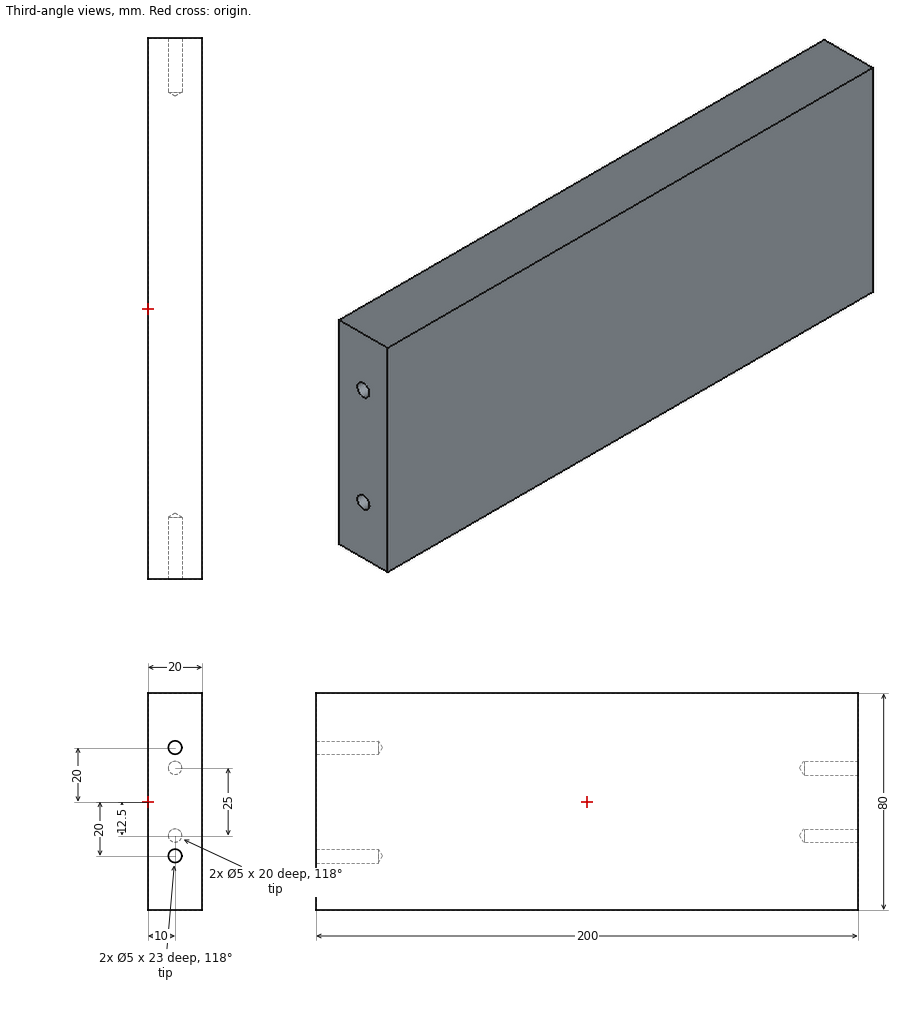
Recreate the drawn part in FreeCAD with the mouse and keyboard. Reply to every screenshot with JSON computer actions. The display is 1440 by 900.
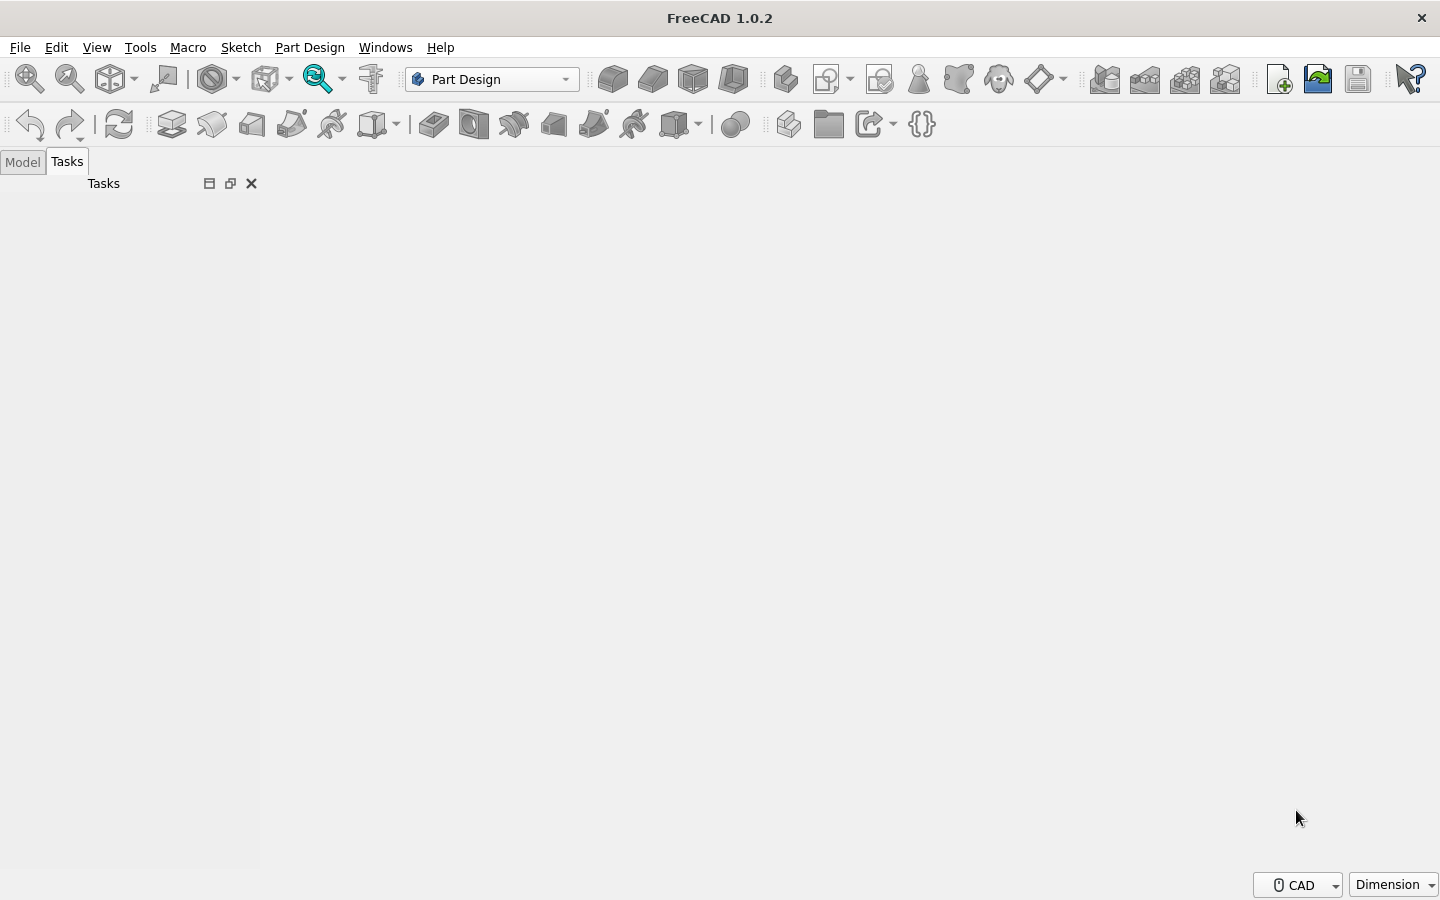
{"action": "left_click", "coordinate": [1278, 80]}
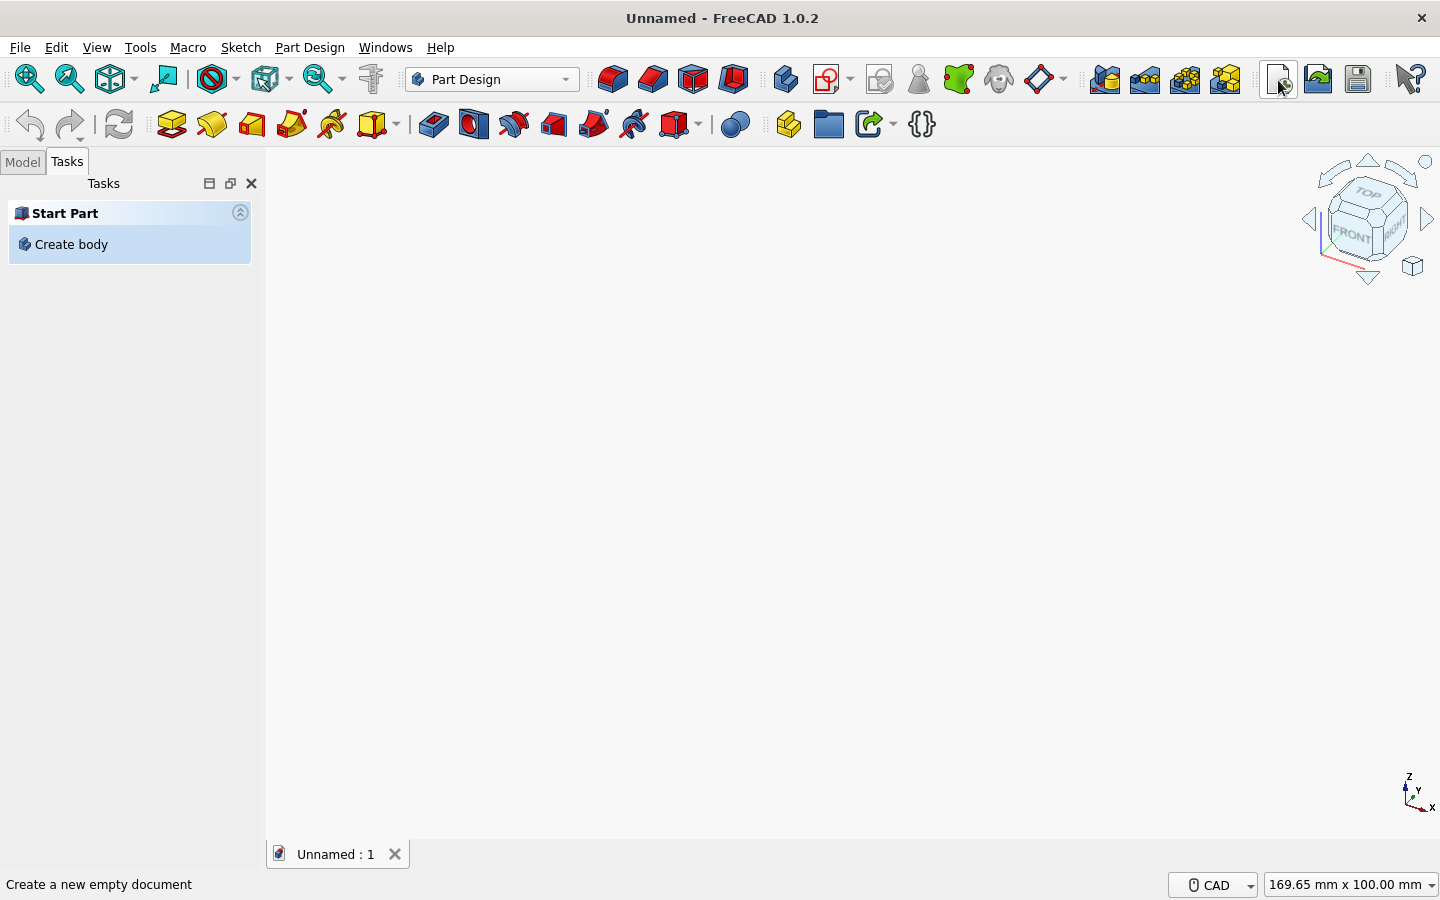
{"action": "left_click", "coordinate": [826, 80]}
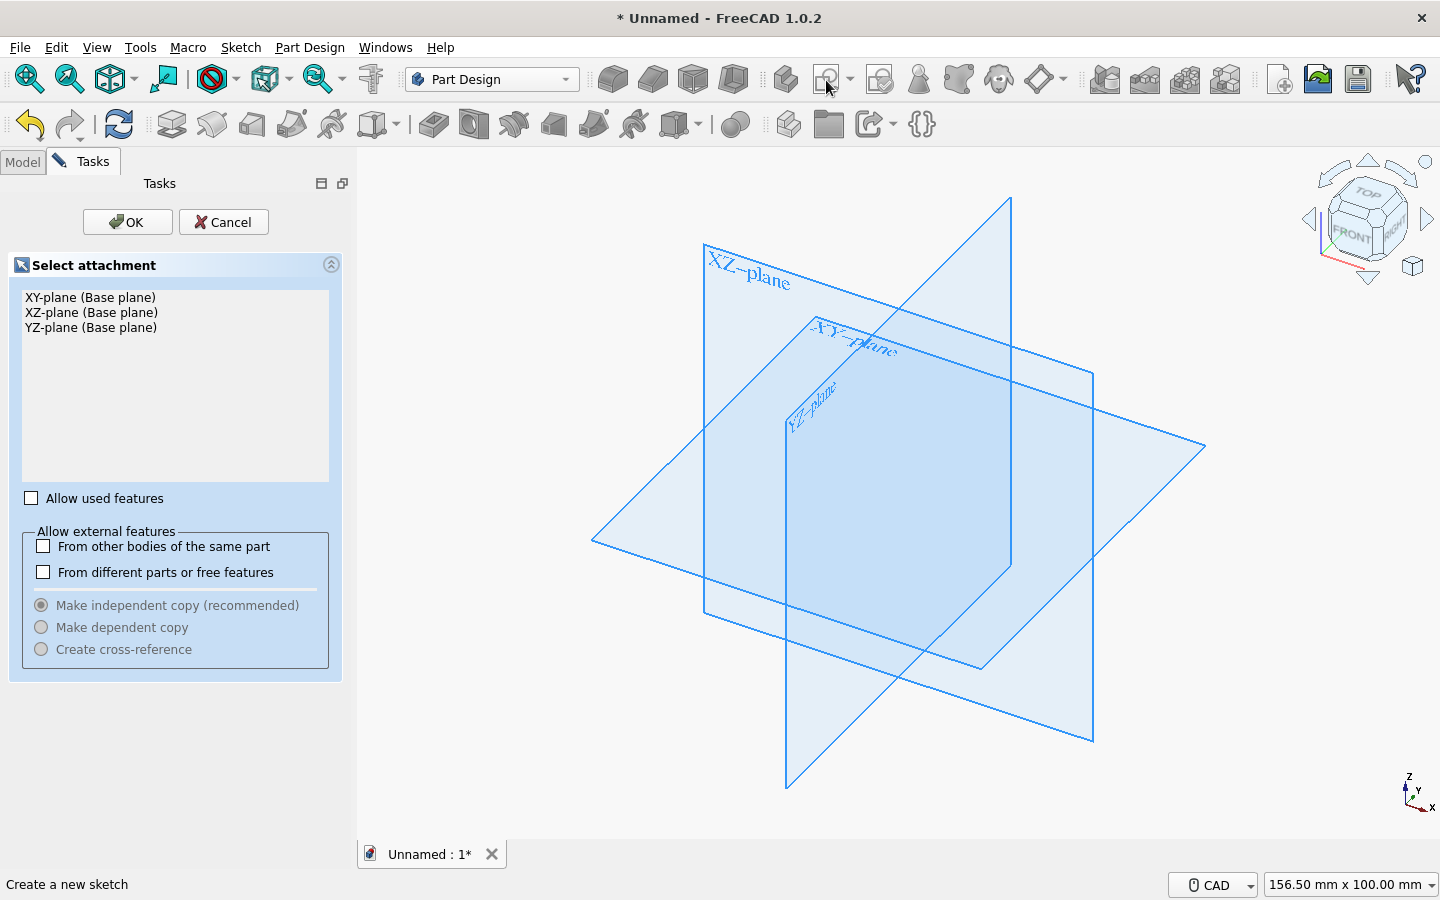
{"action": "left_click", "coordinate": [82, 328]}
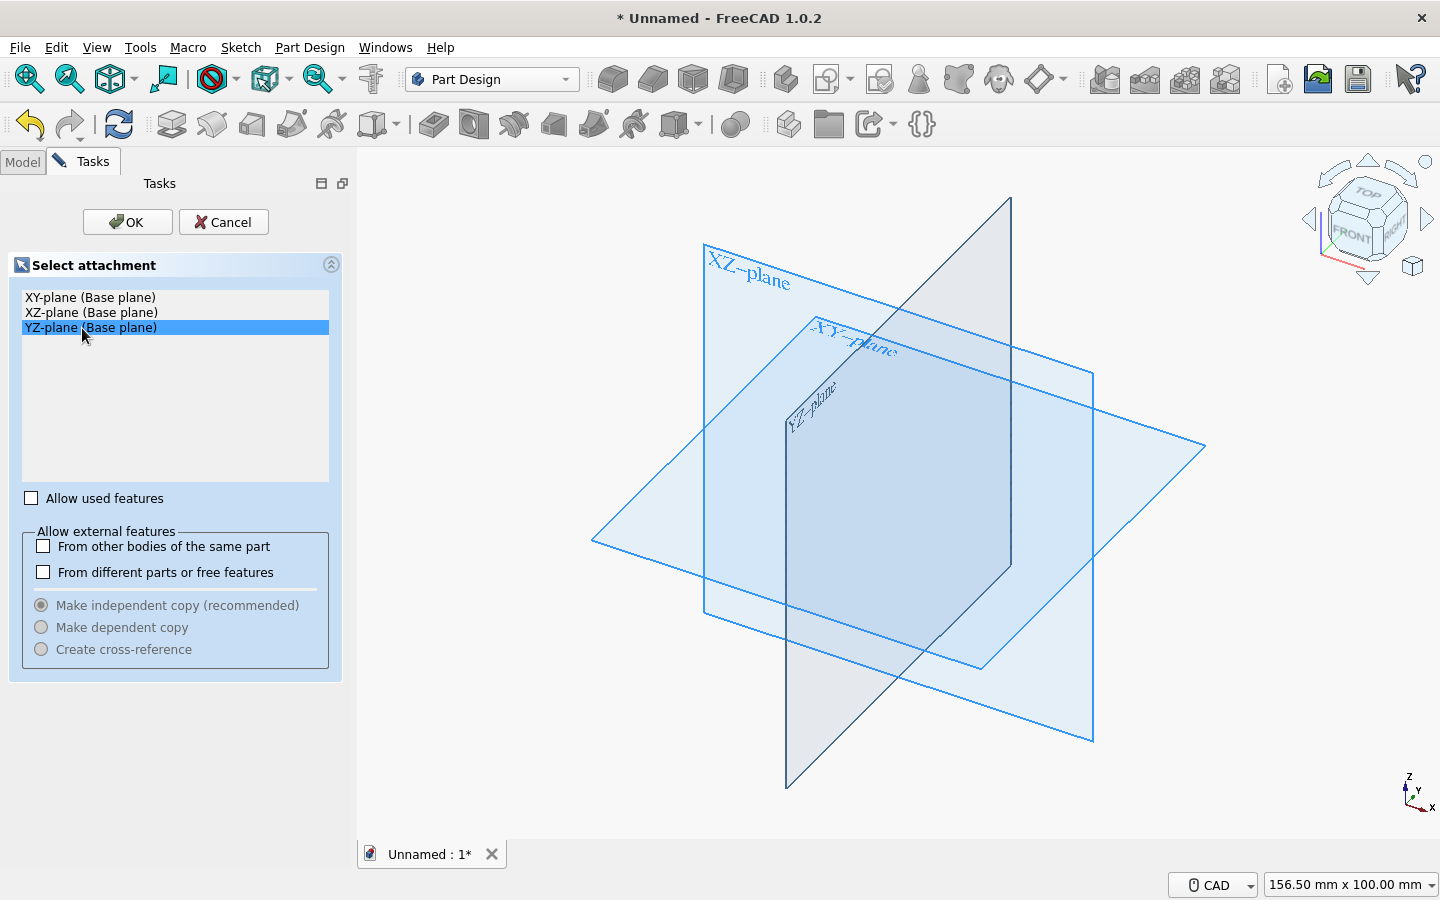
{"action": "left_click", "coordinate": [128, 222]}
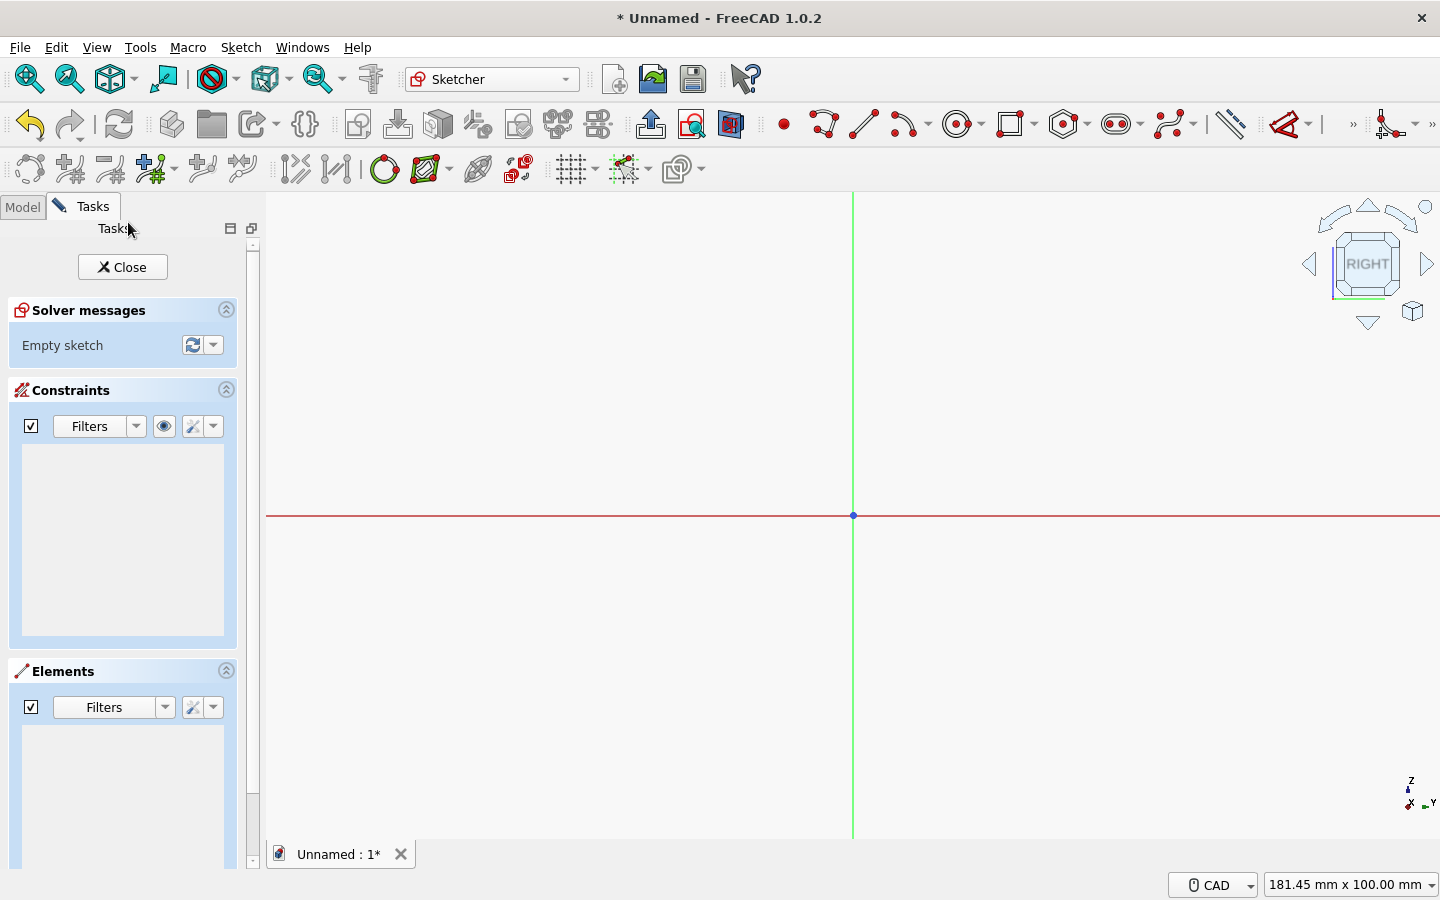
{"action": "scroll", "coordinate": [701, 516], "scroll_direction": "down", "scroll_amount": 3}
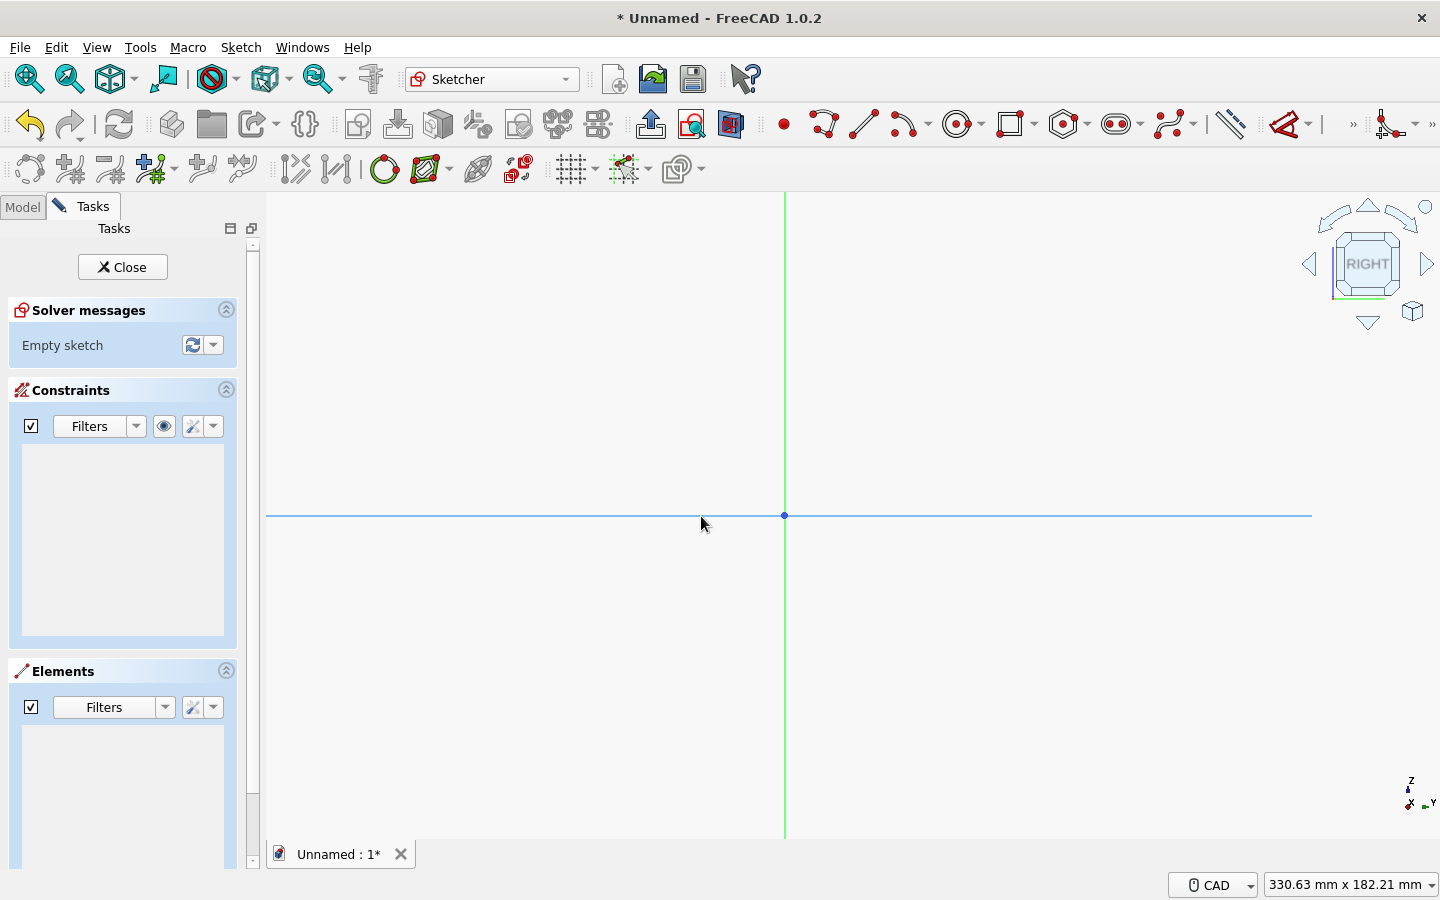
{"action": "key", "text": "g v"}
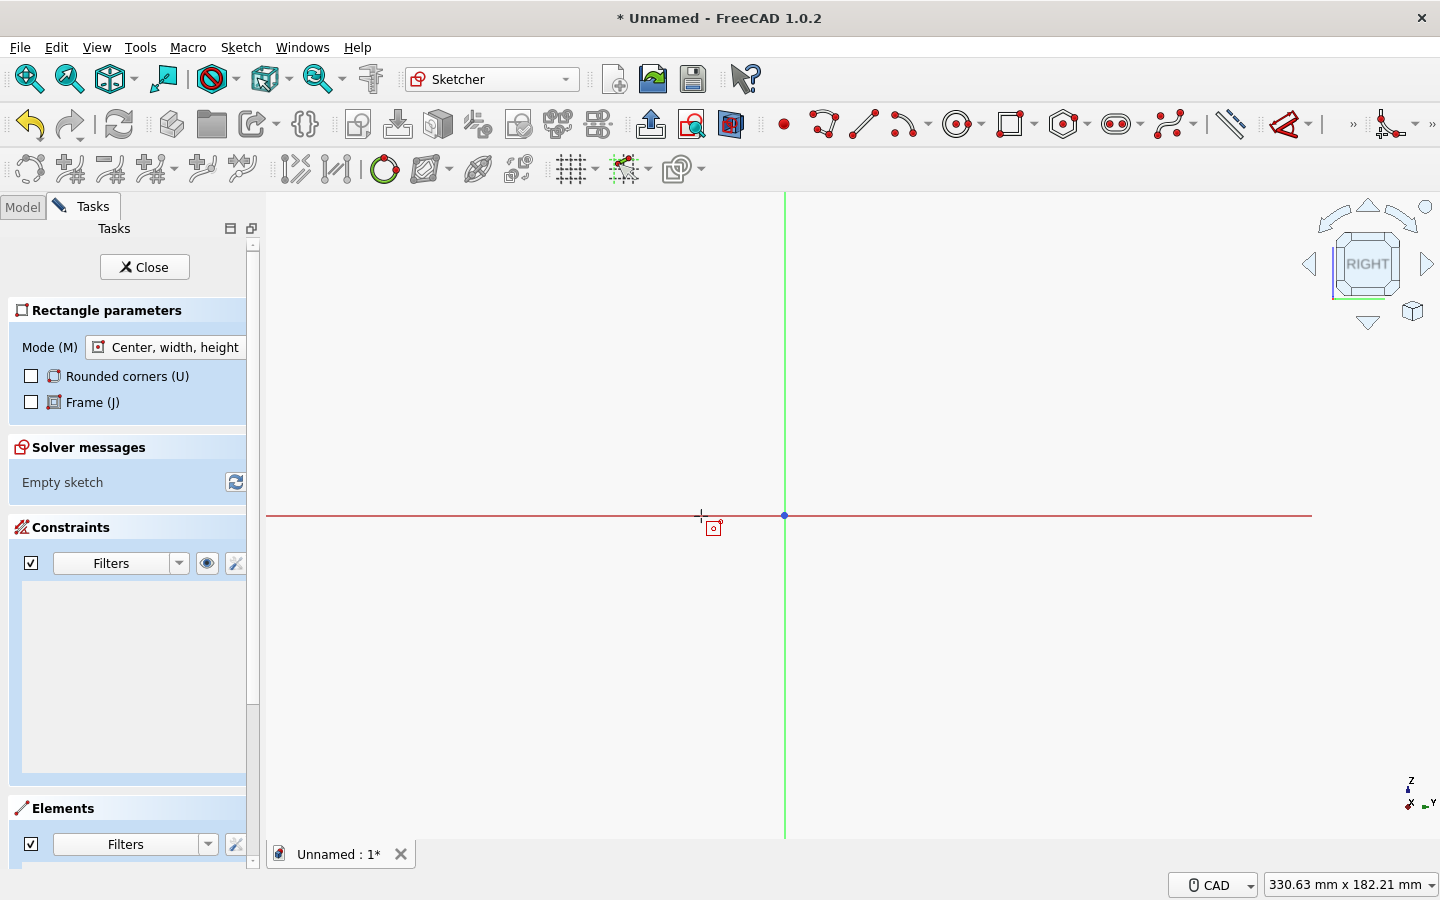
{"action": "left_click", "coordinate": [785, 516]}
{"action": "mouse_move", "coordinate": [1140, 374]}